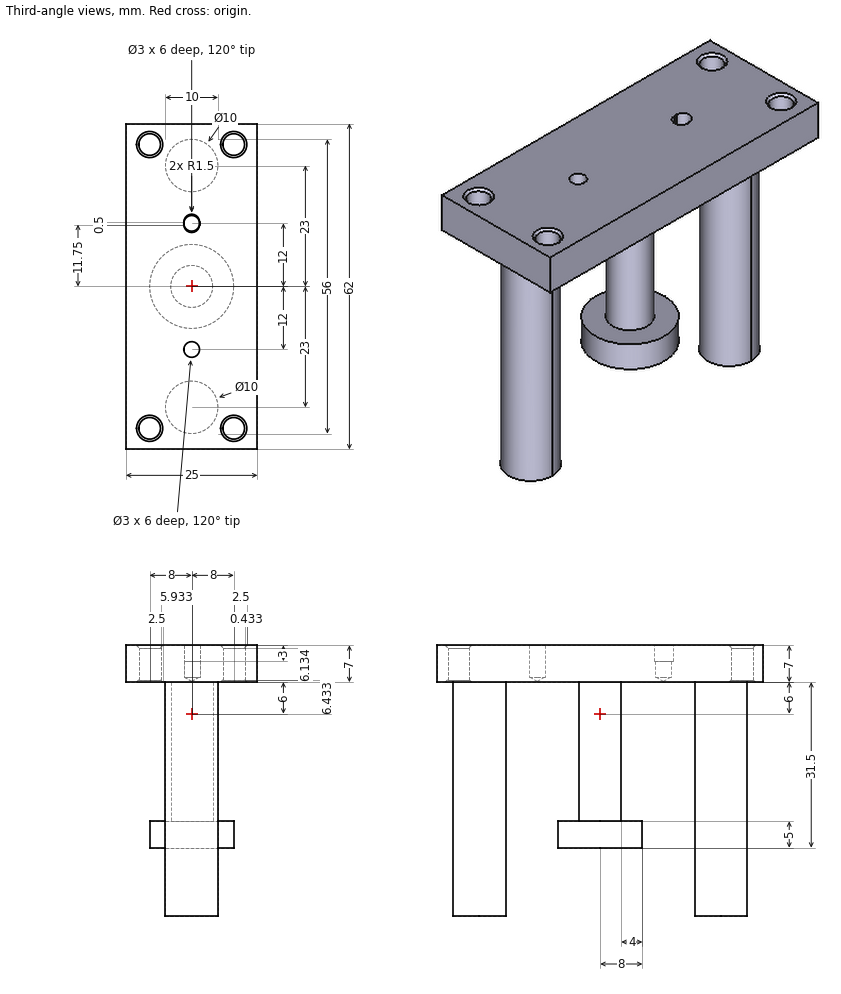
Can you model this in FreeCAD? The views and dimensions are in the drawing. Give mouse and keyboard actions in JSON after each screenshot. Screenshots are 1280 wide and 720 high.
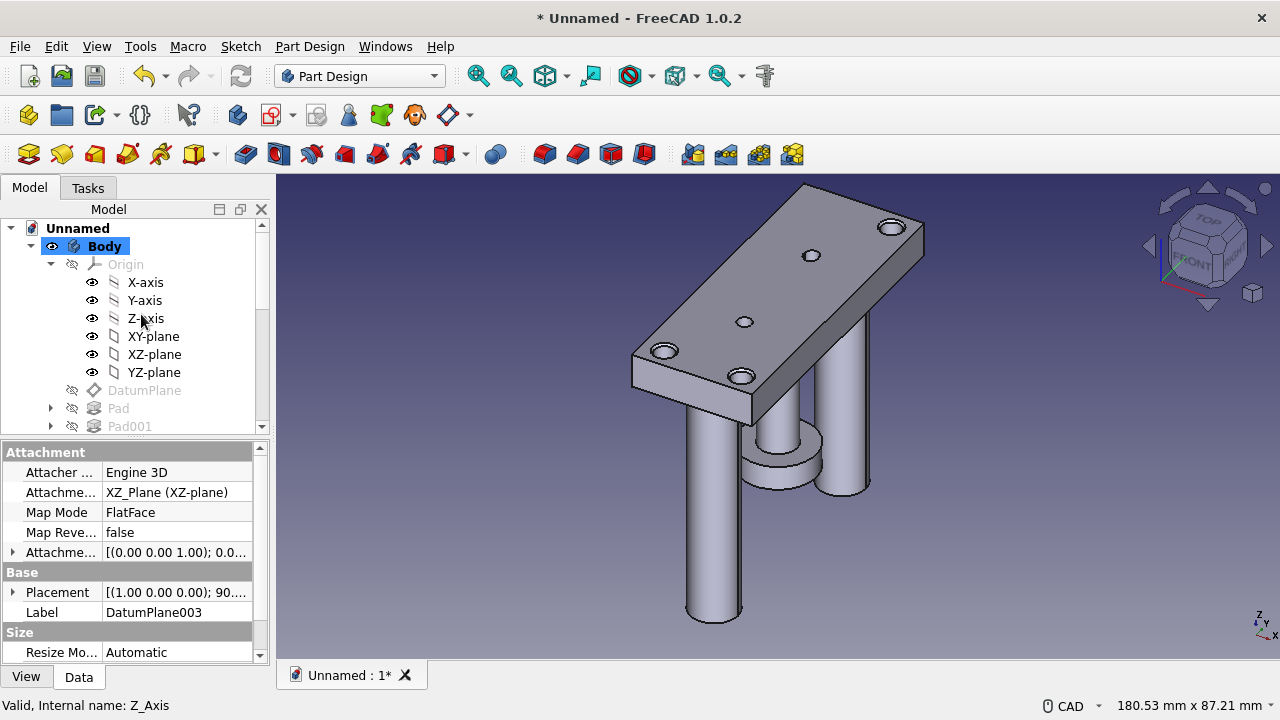
{"action": "left_click", "coordinate": [137, 354]}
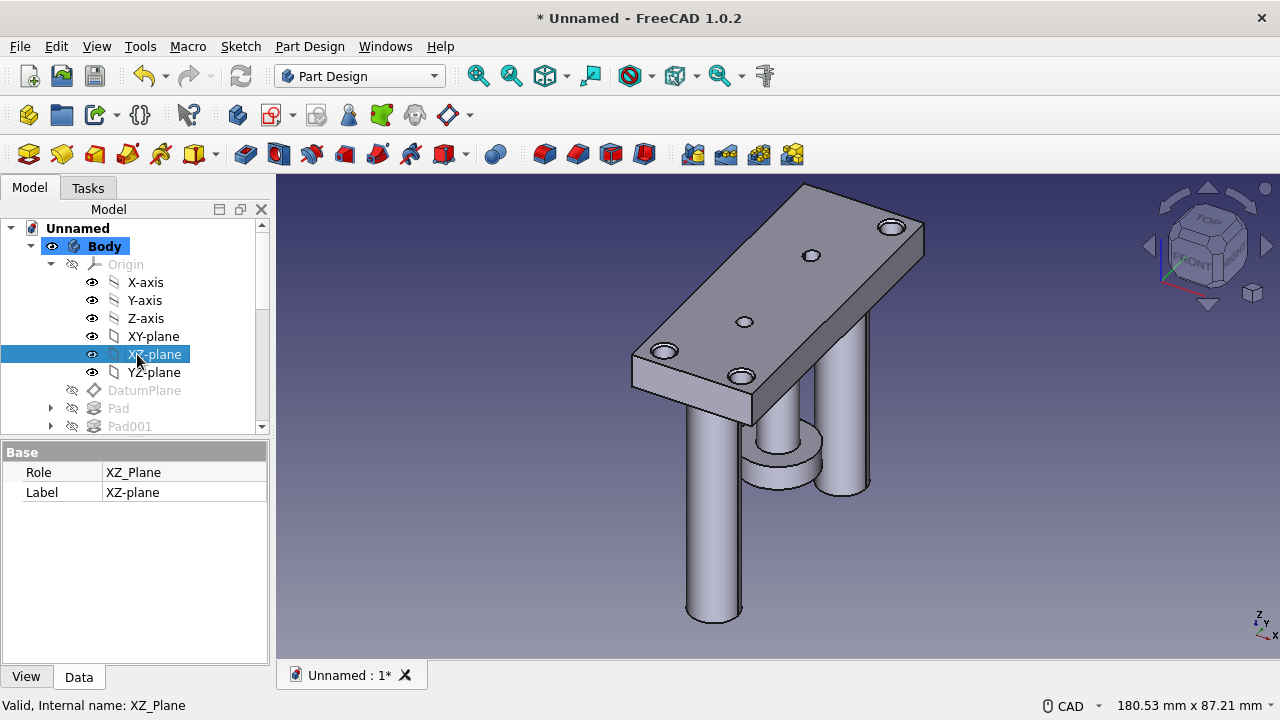
{"action": "left_click", "coordinate": [448, 116]}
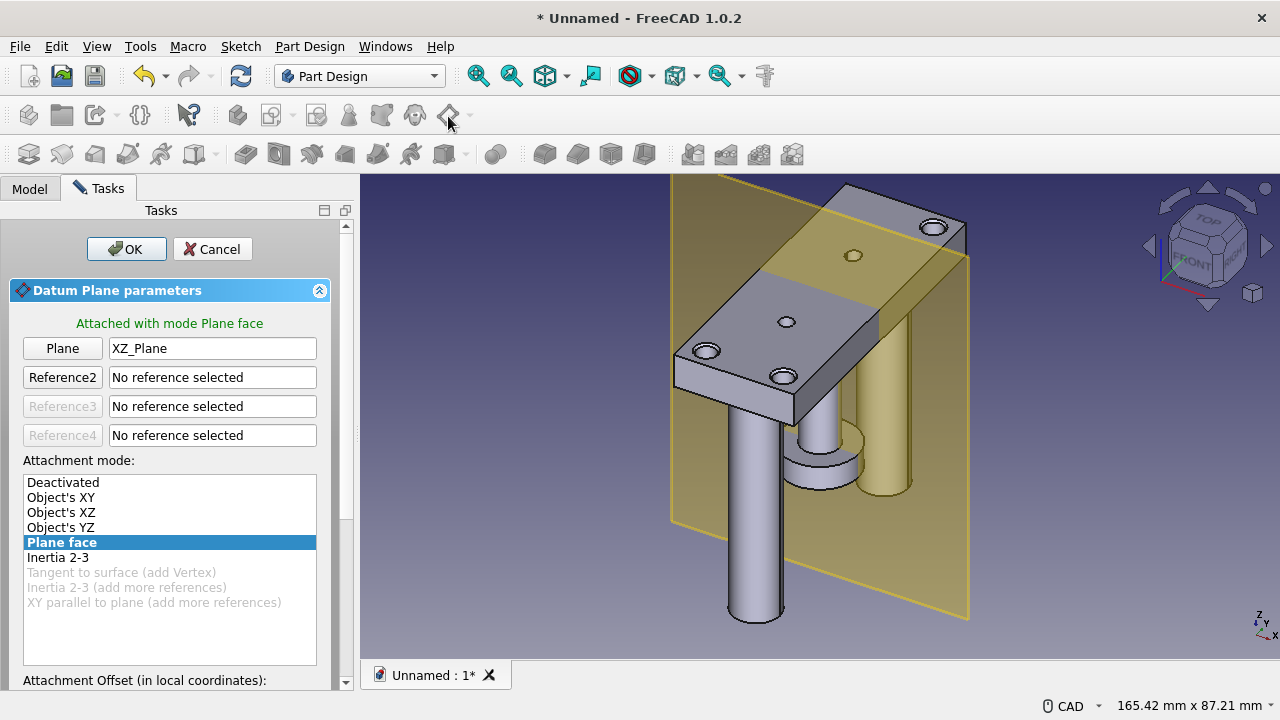
{"action": "scroll", "coordinate": [346, 455], "scroll_direction": "down", "scroll_amount": 3}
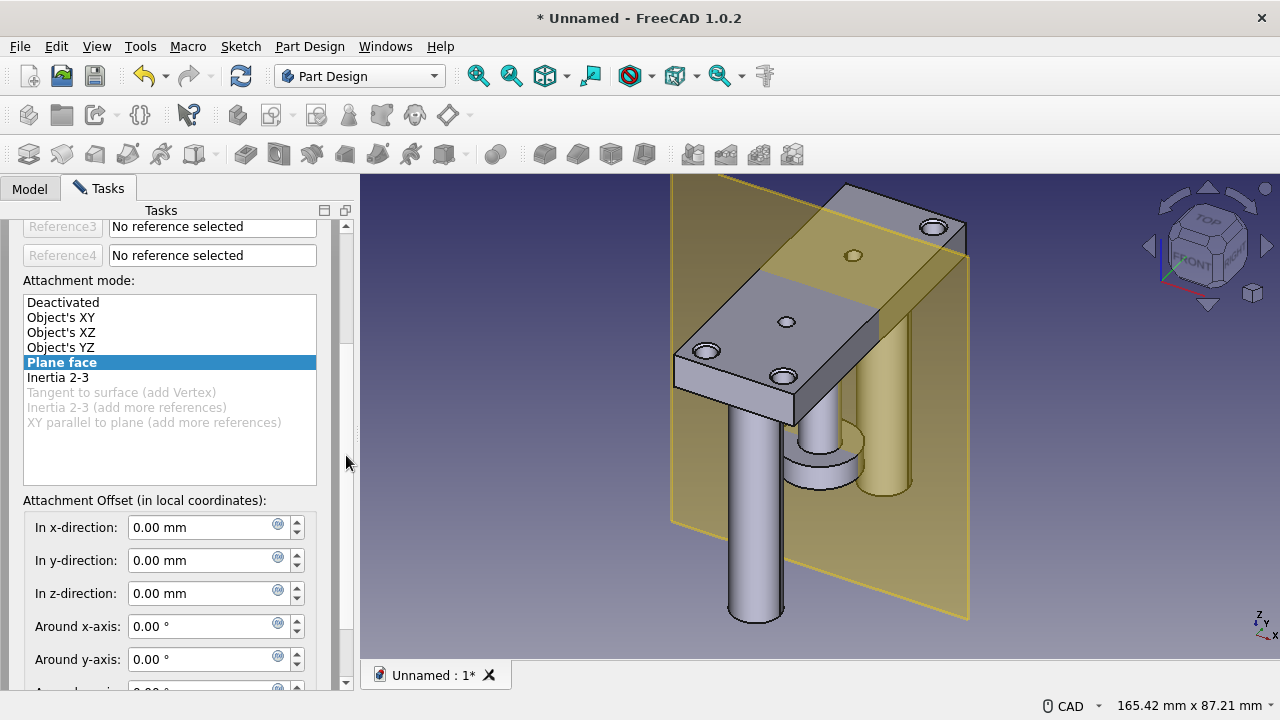
{"action": "triple_click", "coordinate": [210, 594]}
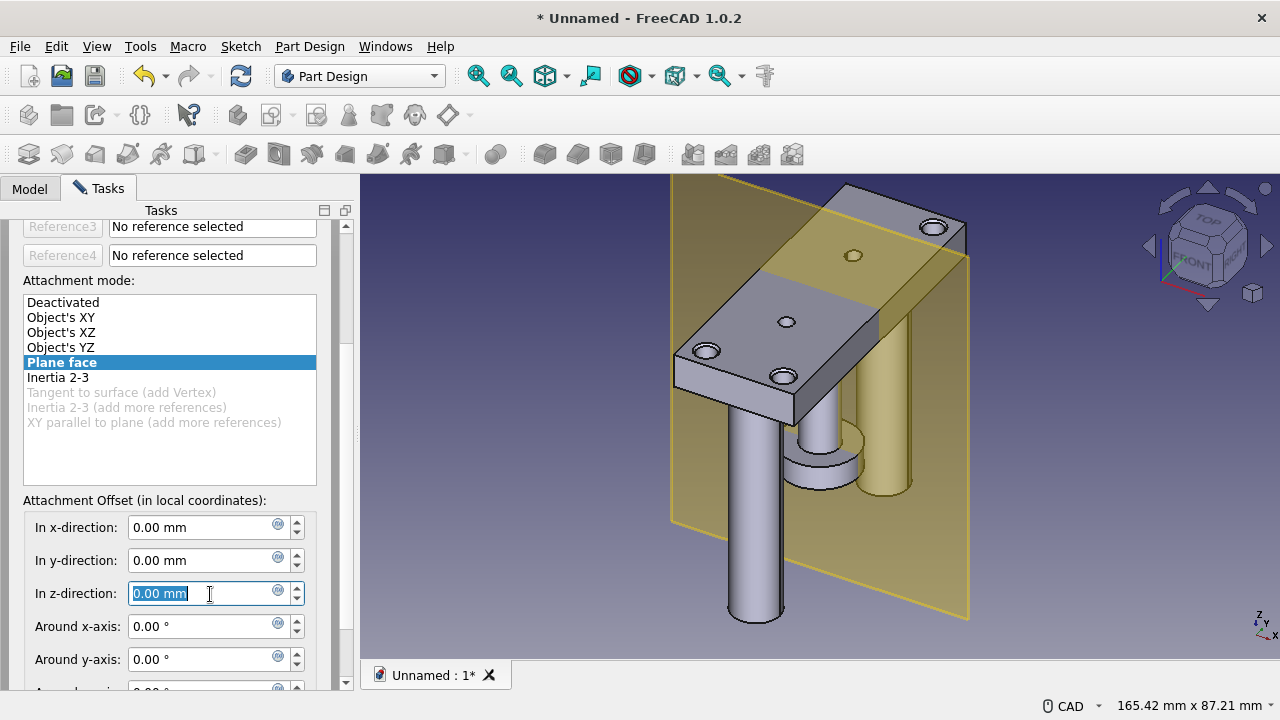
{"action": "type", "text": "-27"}
{"action": "key", "text": "Tab"}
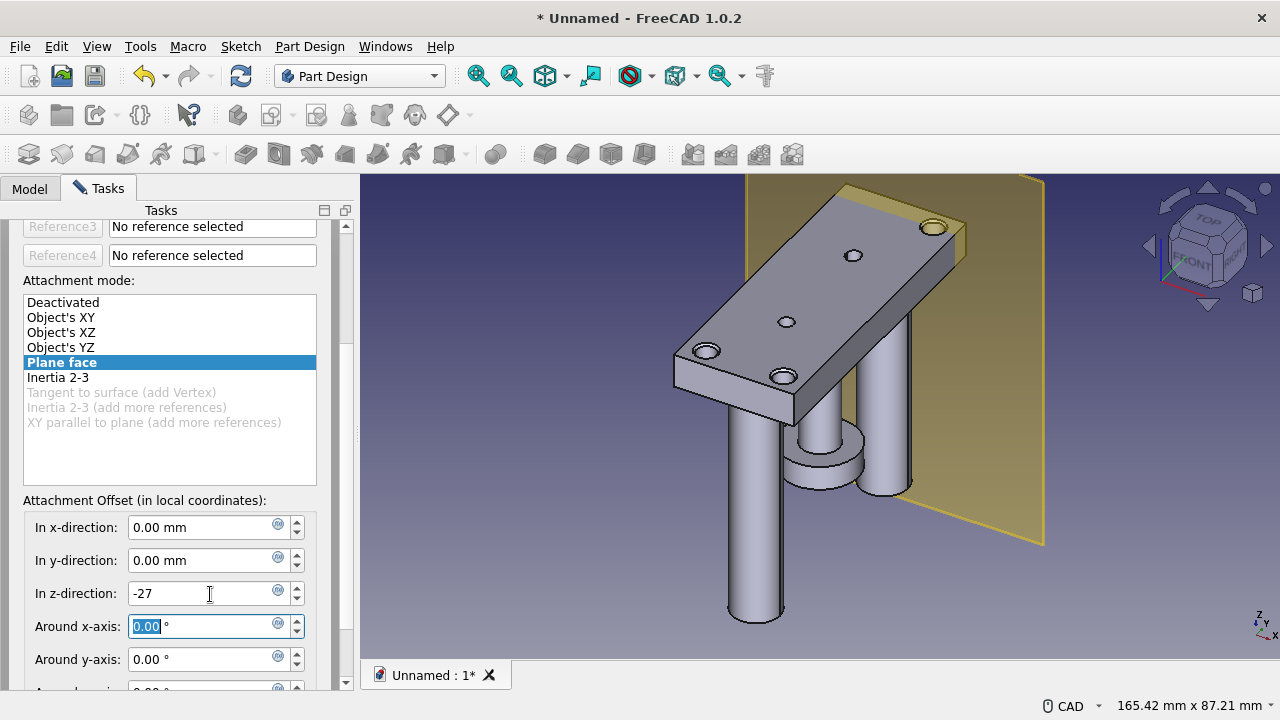
{"action": "scroll", "coordinate": [346, 455], "scroll_direction": "up", "scroll_amount": 4}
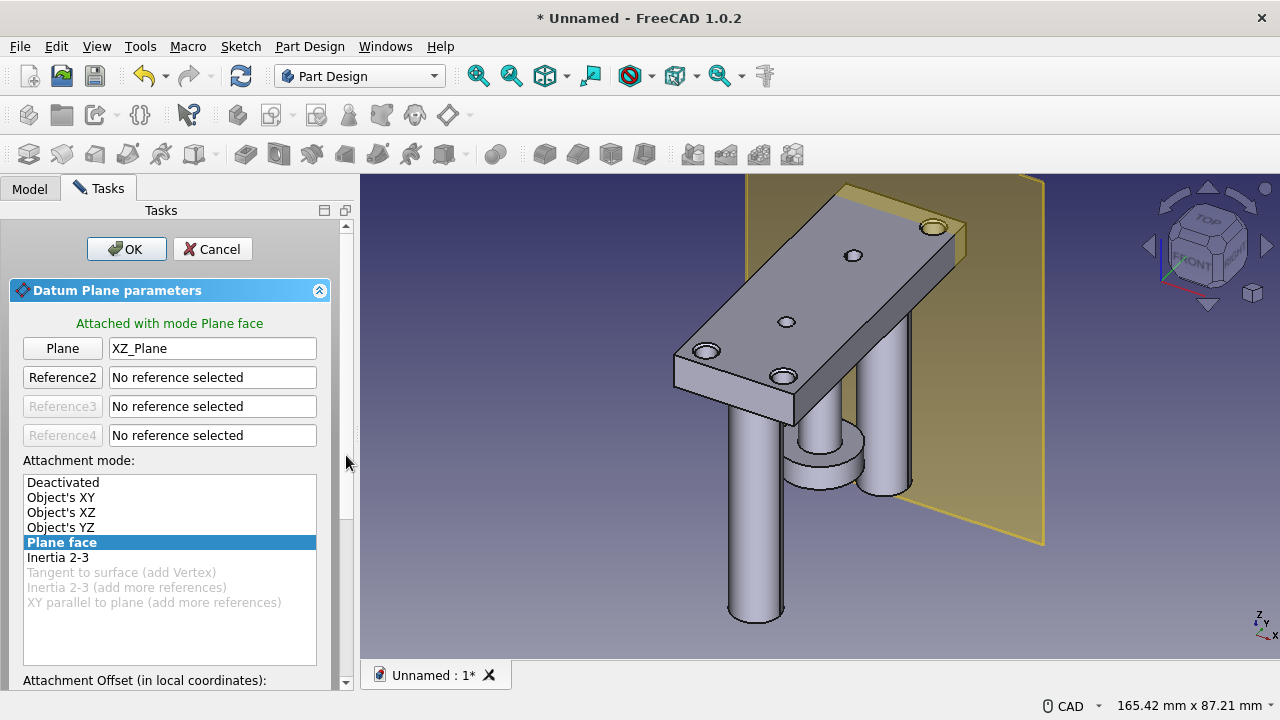
{"action": "left_click", "coordinate": [127, 249]}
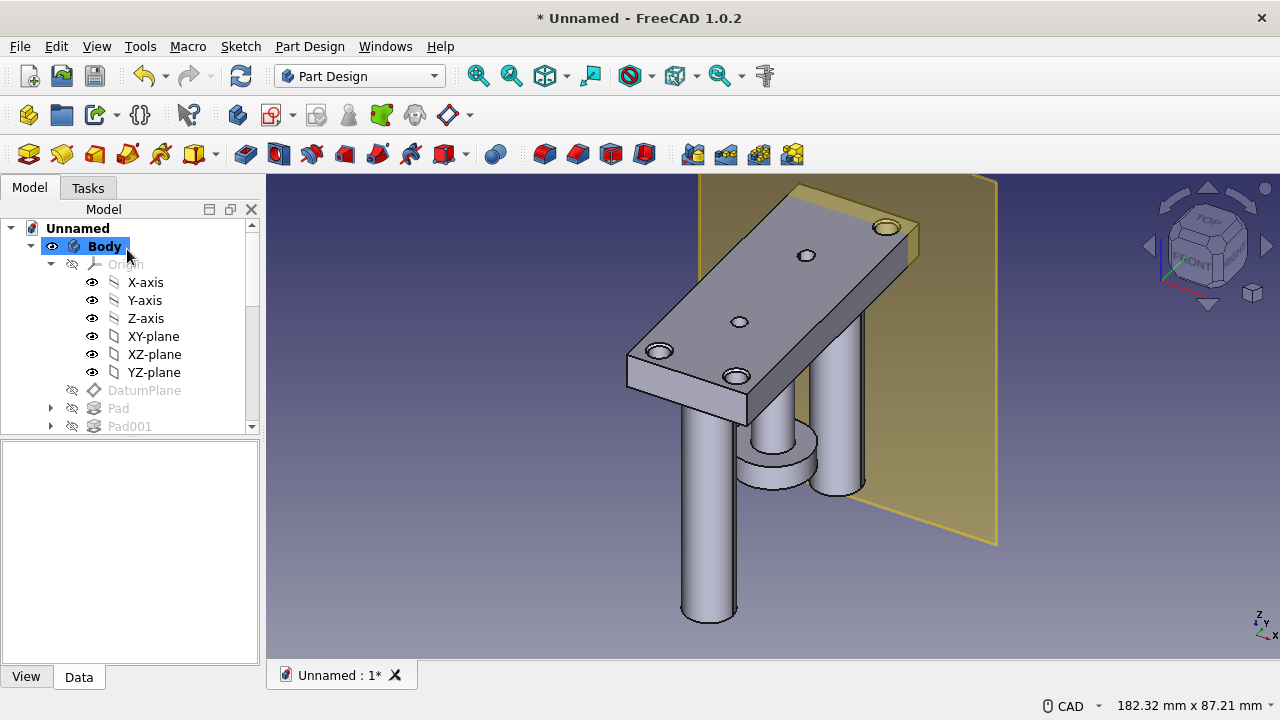
{"action": "scroll", "coordinate": [101, 332], "scroll_direction": "down", "scroll_amount": 3}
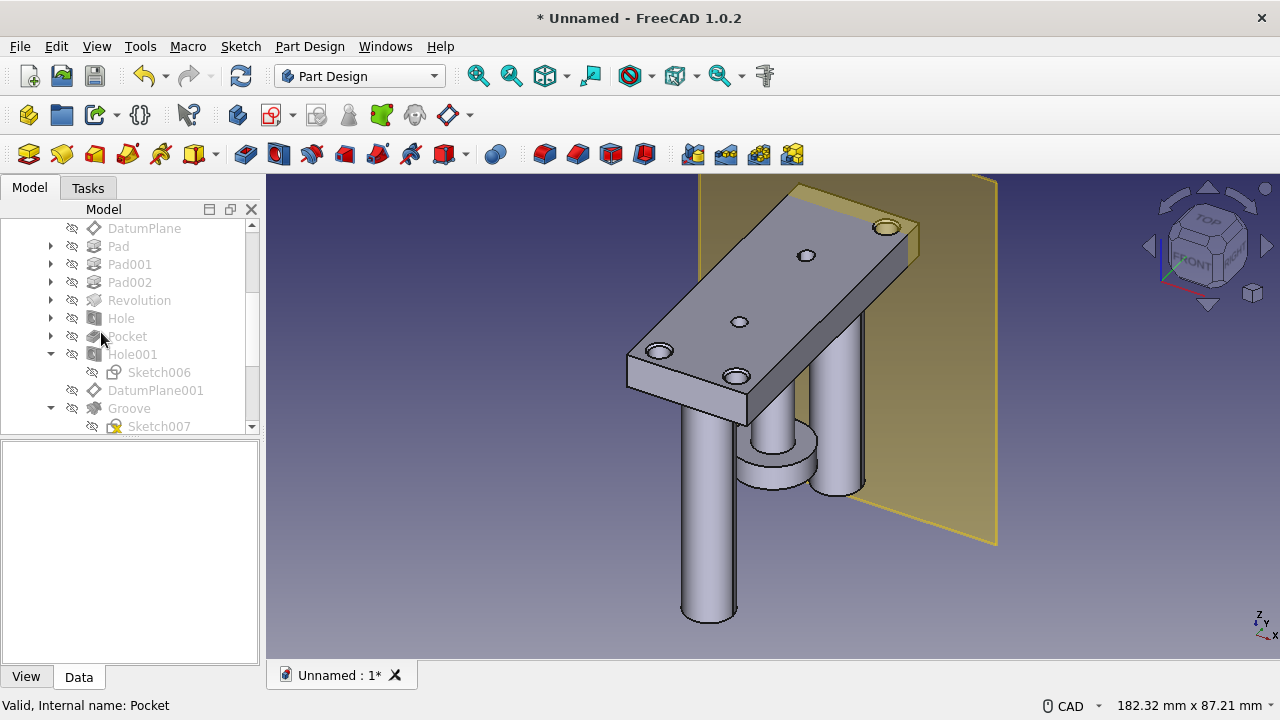
{"action": "scroll", "coordinate": [141, 332], "scroll_direction": "up", "scroll_amount": 15}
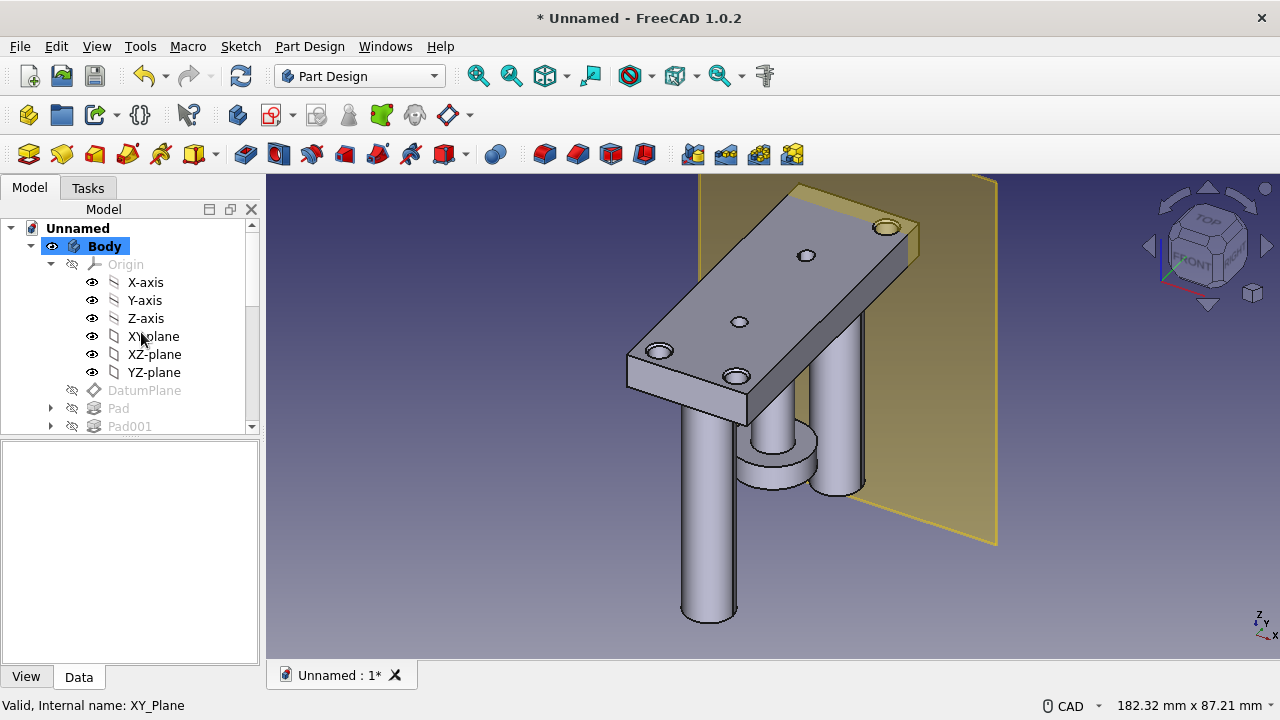
{"action": "scroll", "coordinate": [101, 332], "scroll_direction": "down", "scroll_amount": 6}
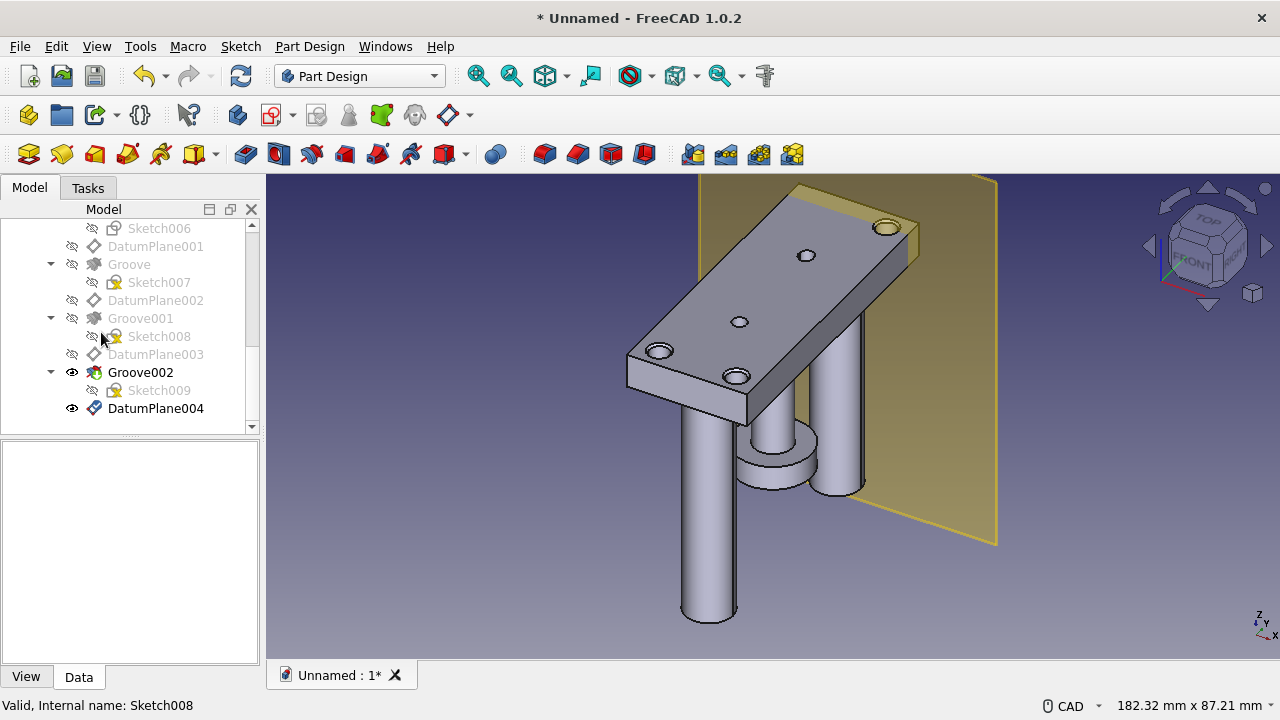
{"action": "left_click", "coordinate": [117, 408]}